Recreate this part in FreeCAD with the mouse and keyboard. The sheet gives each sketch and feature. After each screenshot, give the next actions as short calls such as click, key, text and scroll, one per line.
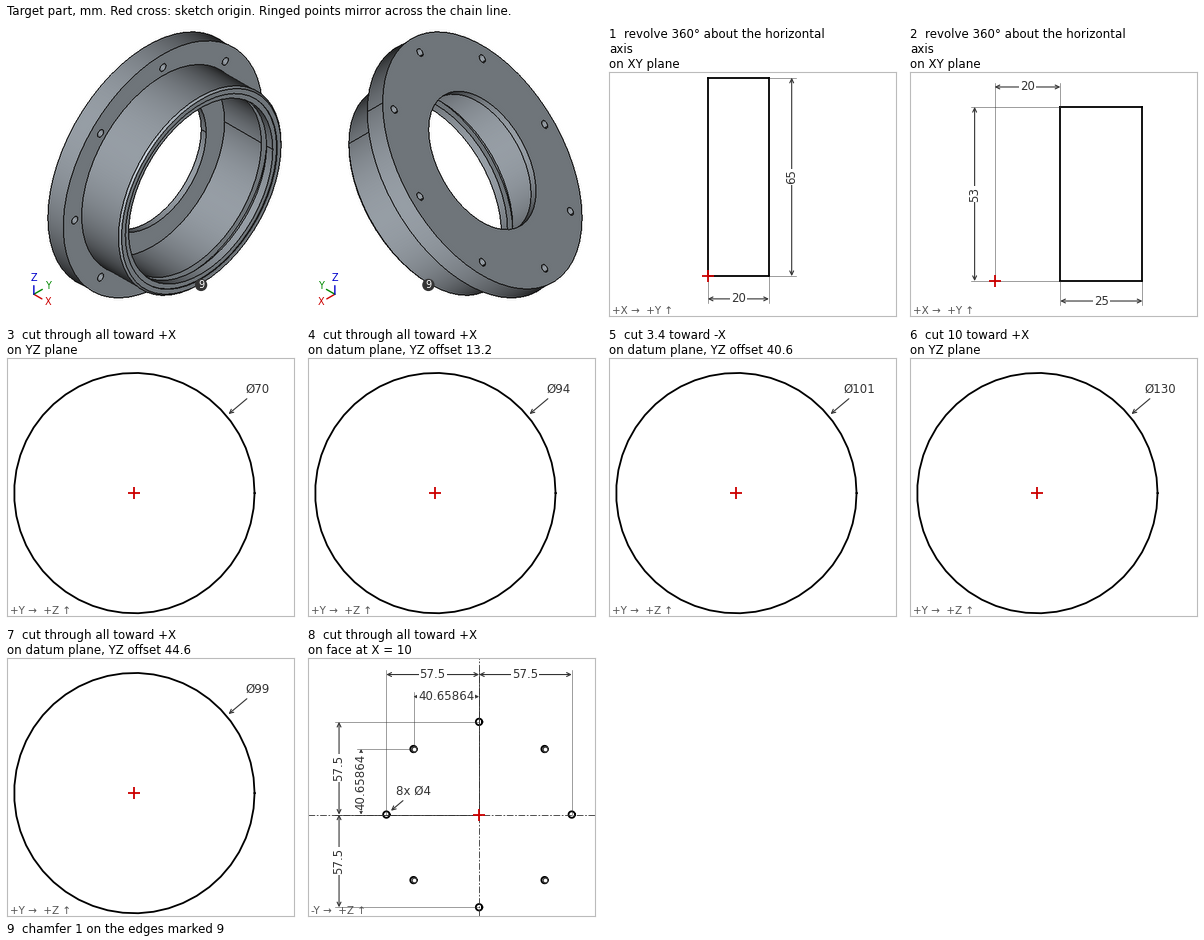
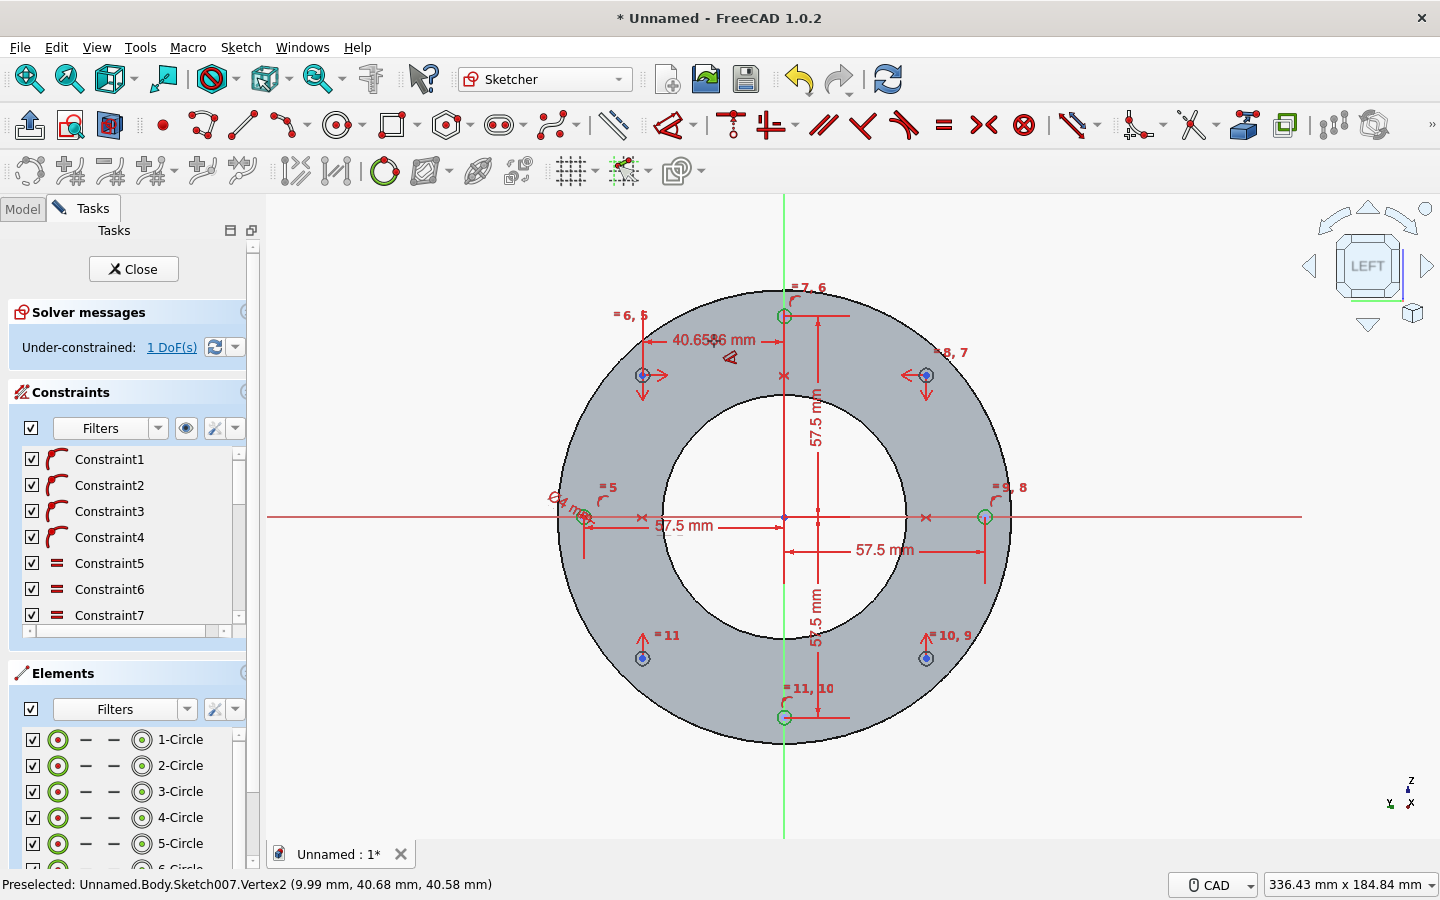
click(643, 375)
click(609, 446)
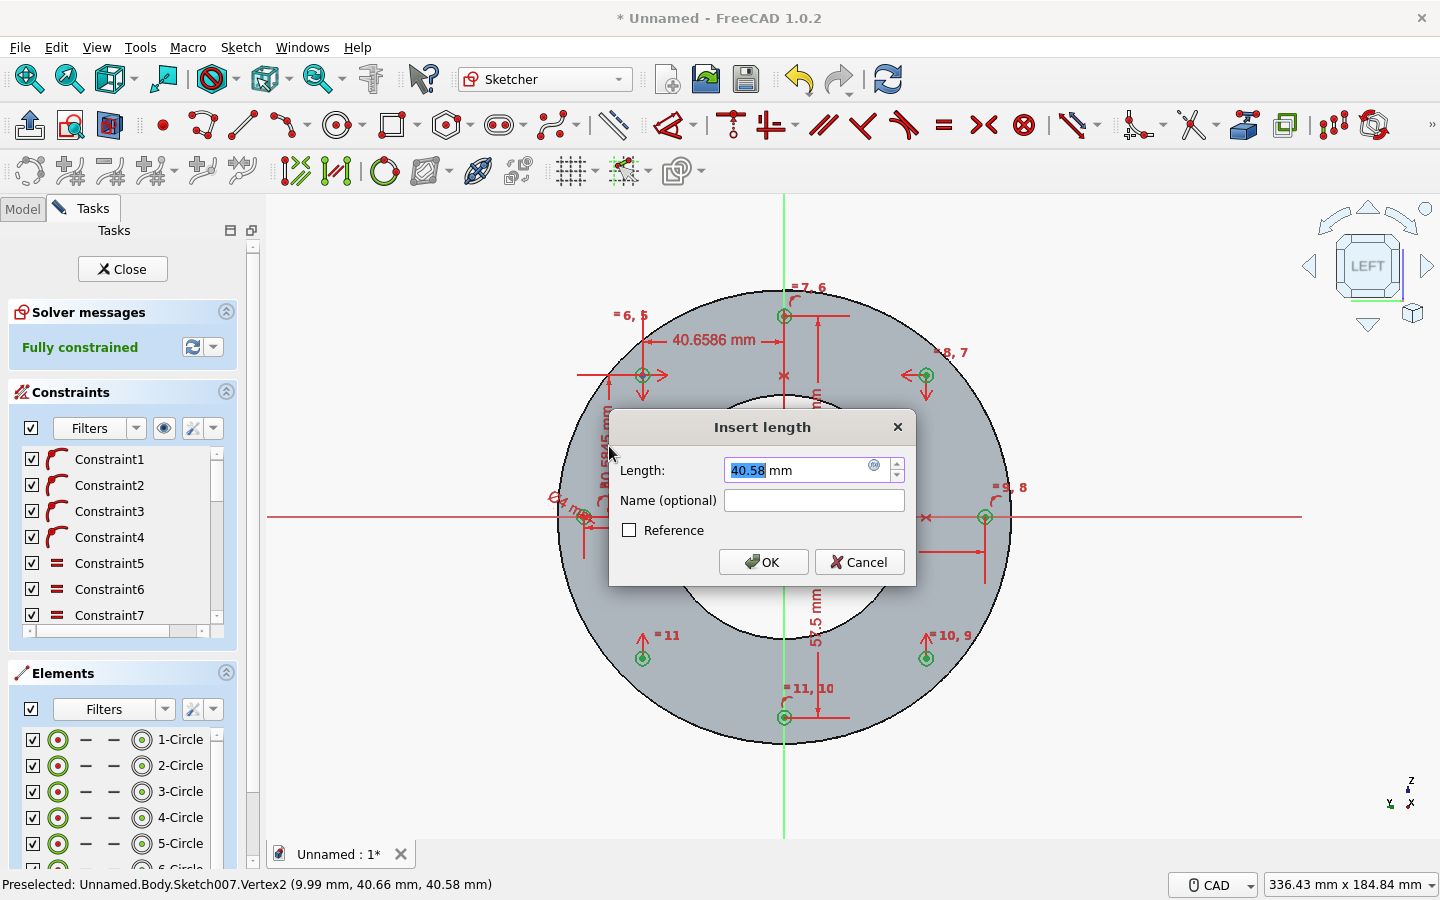
text(40.65864)
key(Return)
key(Escape)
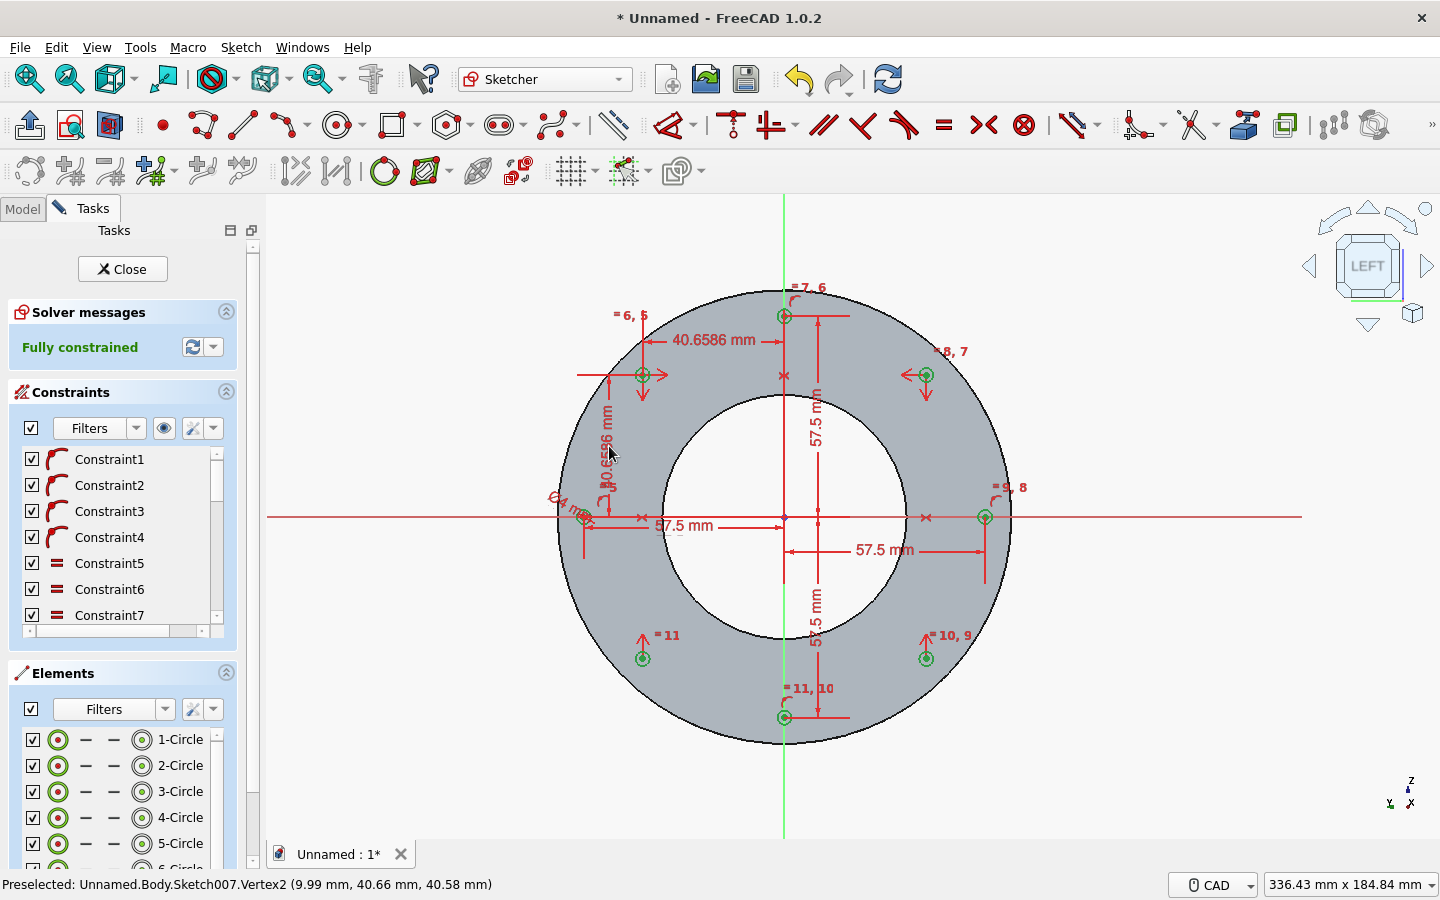
click(123, 269)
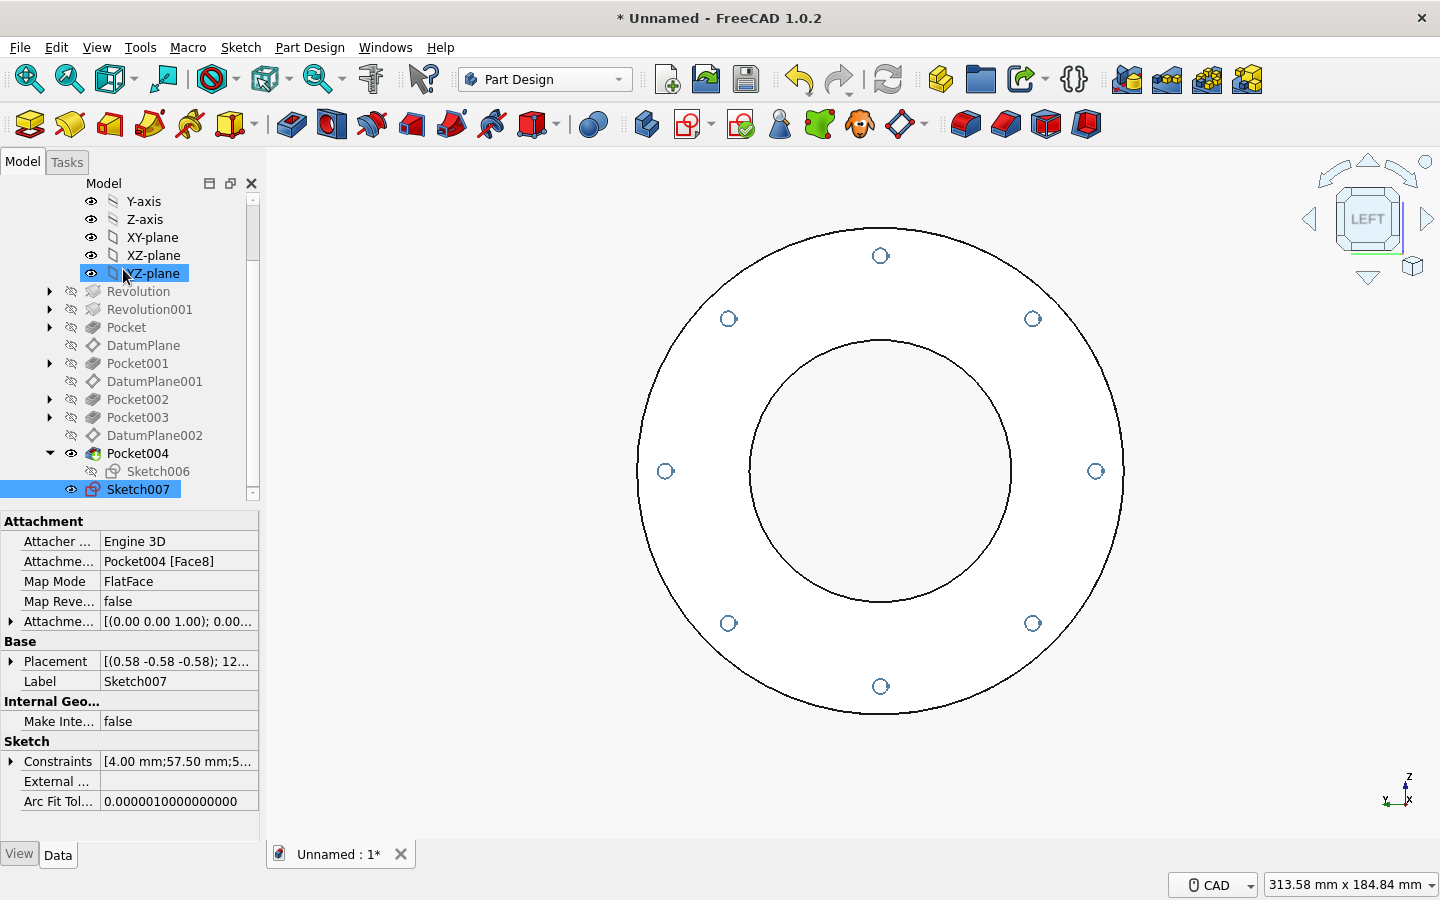
click(292, 124)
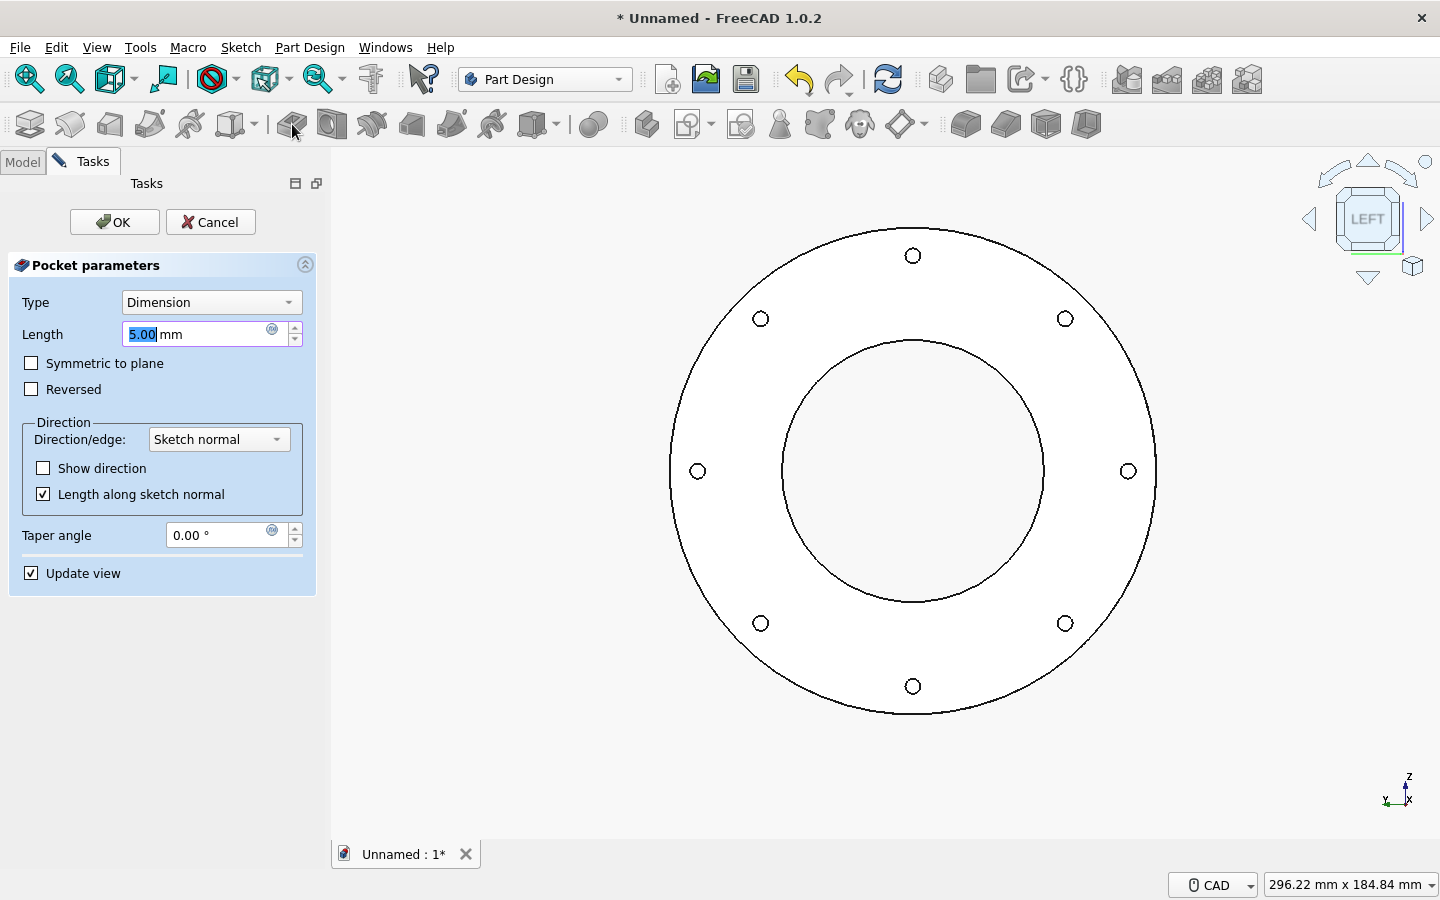
click(212, 302)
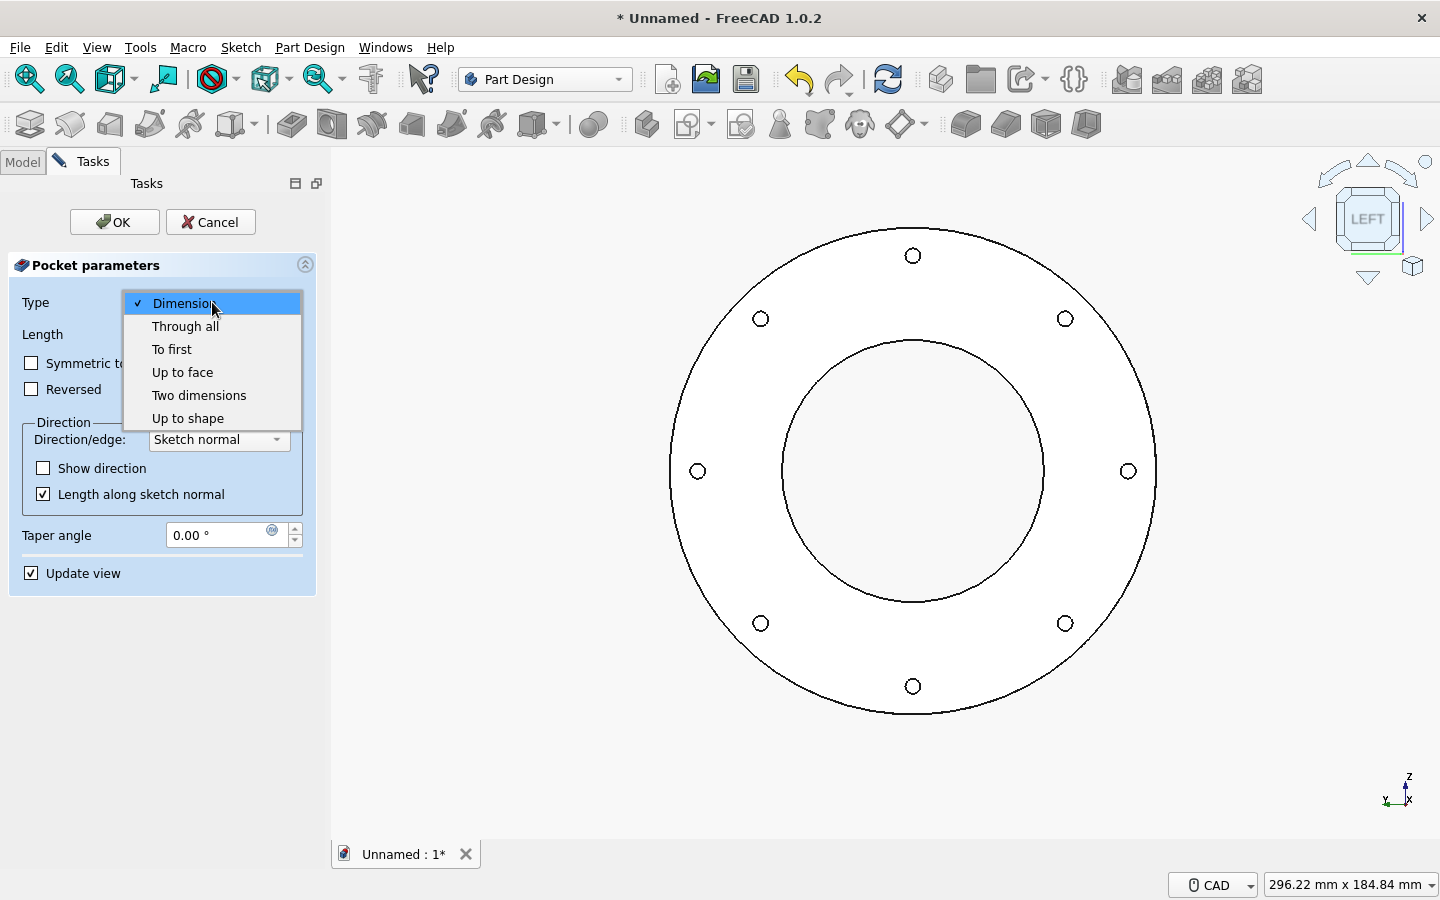
click(212, 326)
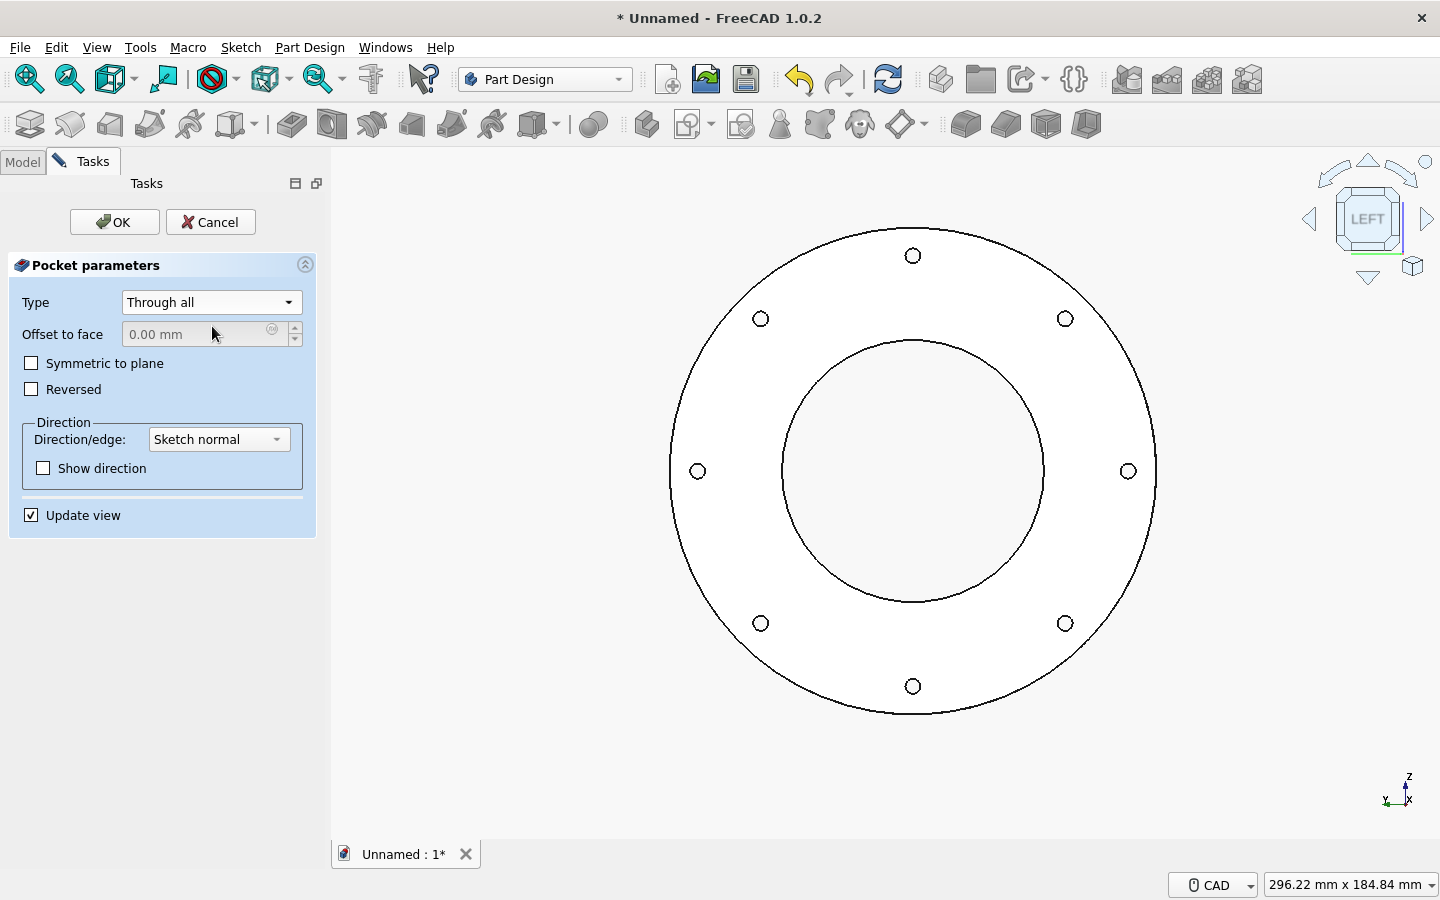
click(115, 222)